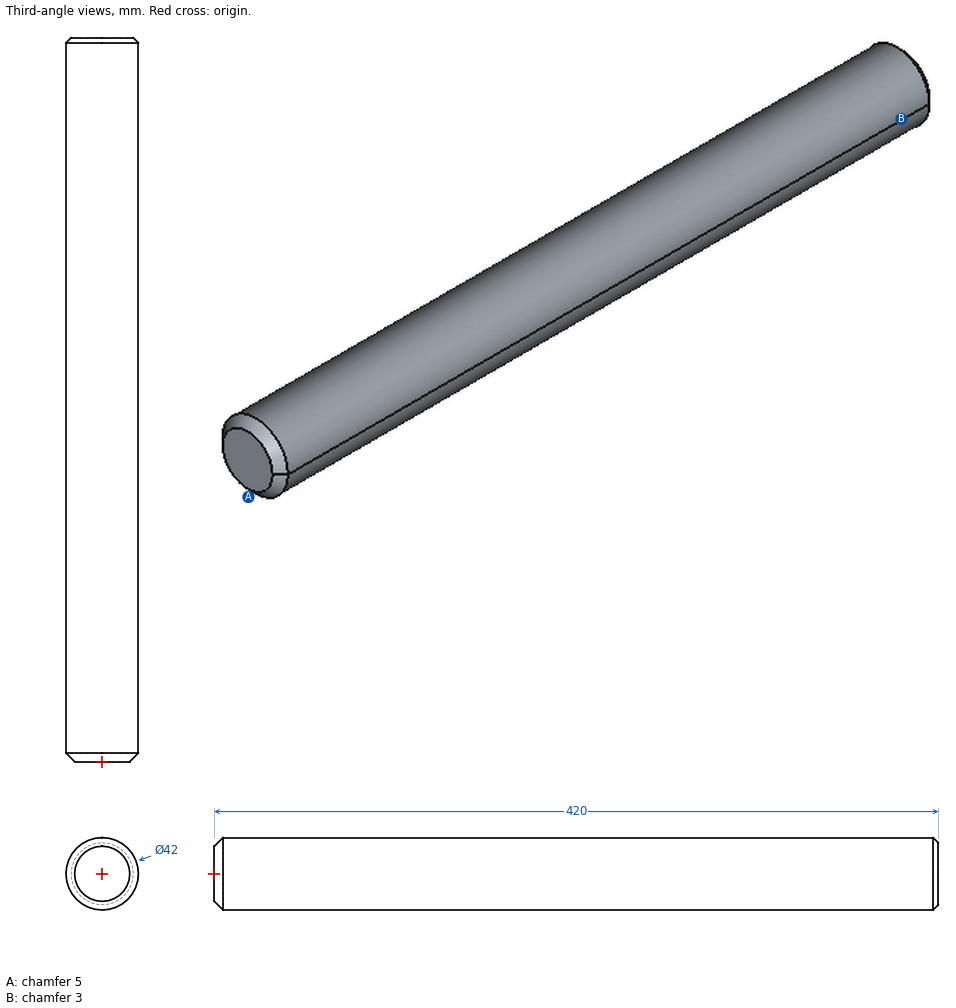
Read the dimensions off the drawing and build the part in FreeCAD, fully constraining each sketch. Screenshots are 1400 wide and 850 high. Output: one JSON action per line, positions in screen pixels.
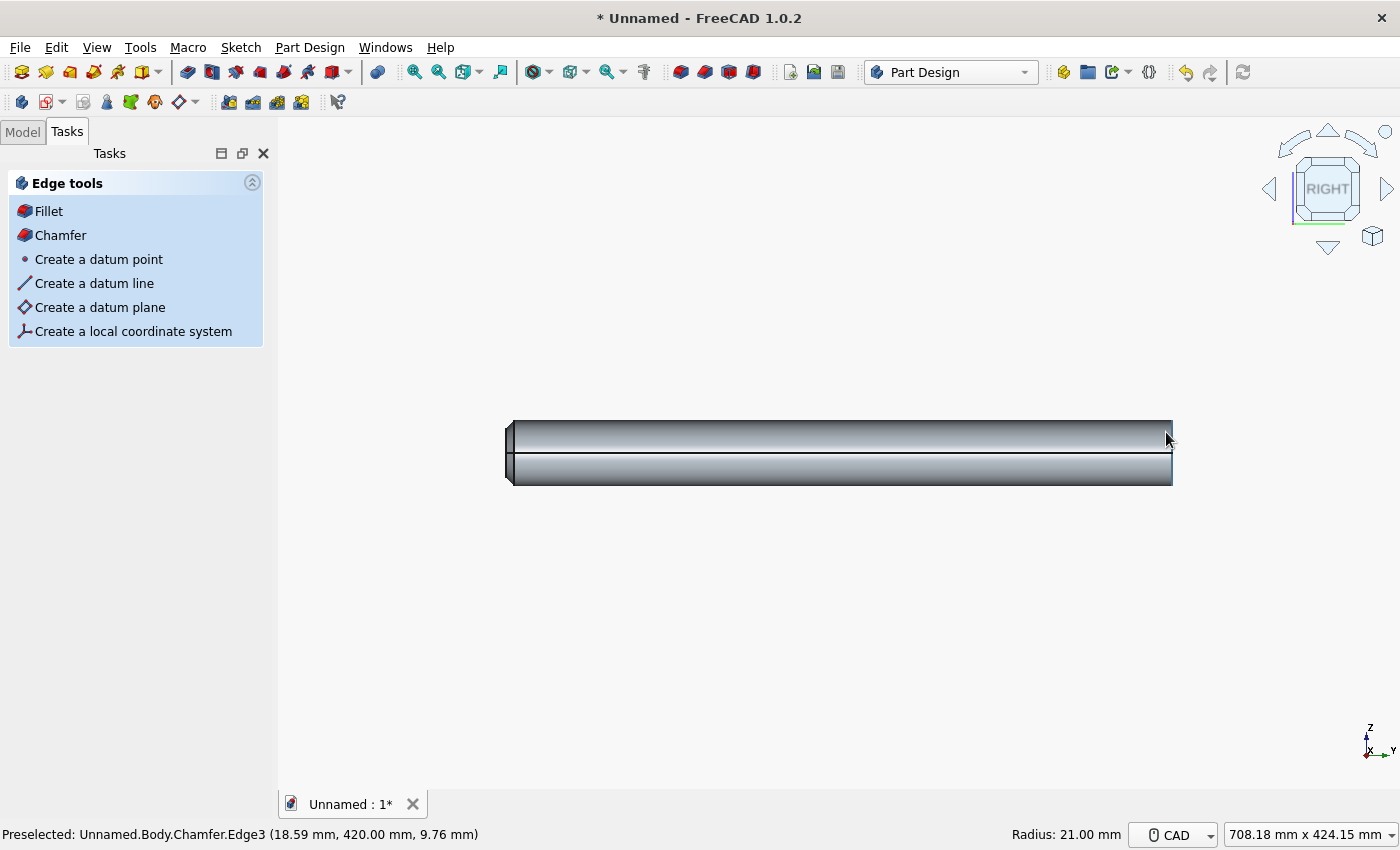
{"action": "left_click", "coordinate": [706, 72]}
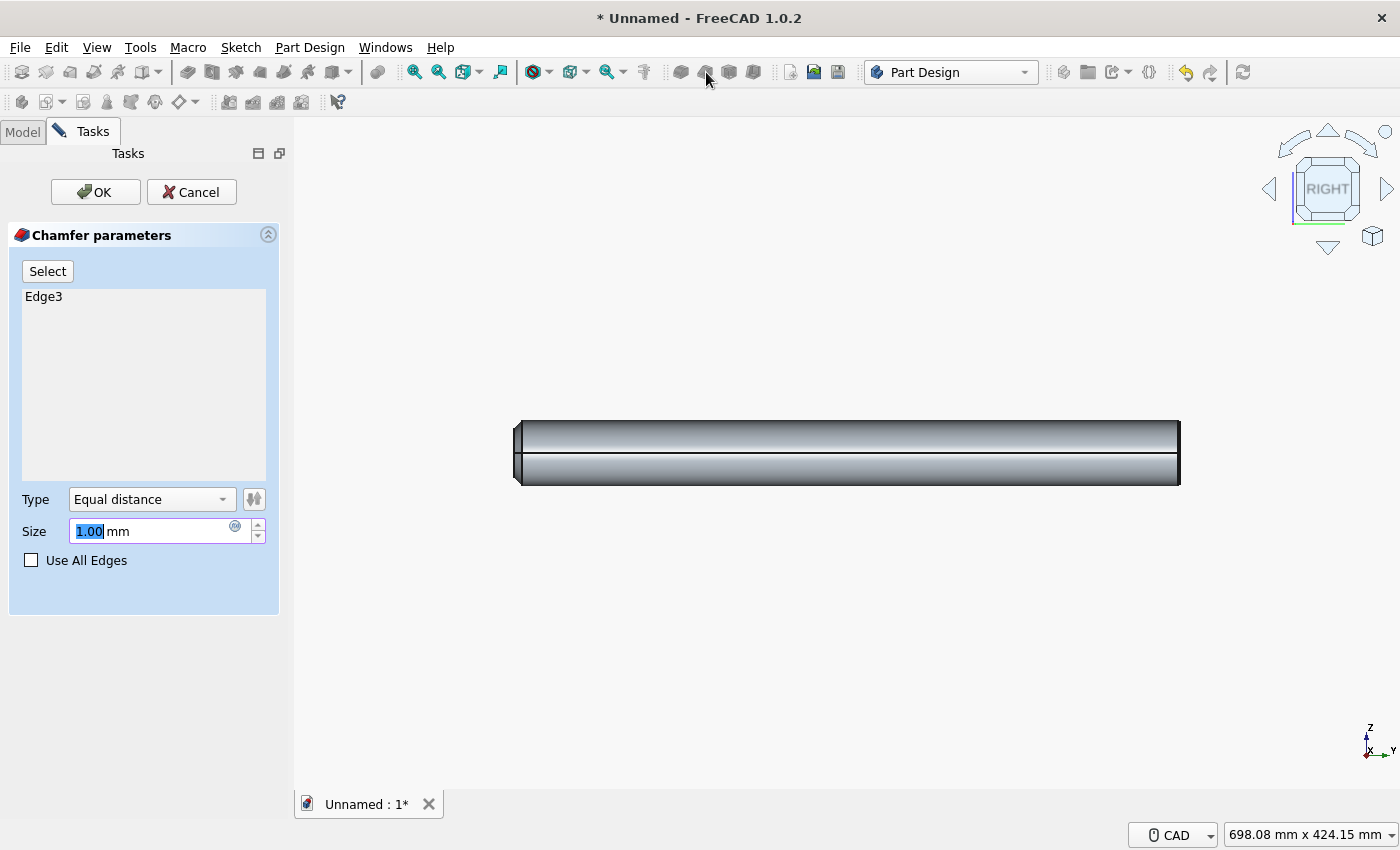
{"action": "type", "text": "3"}
{"action": "key", "text": "Tab"}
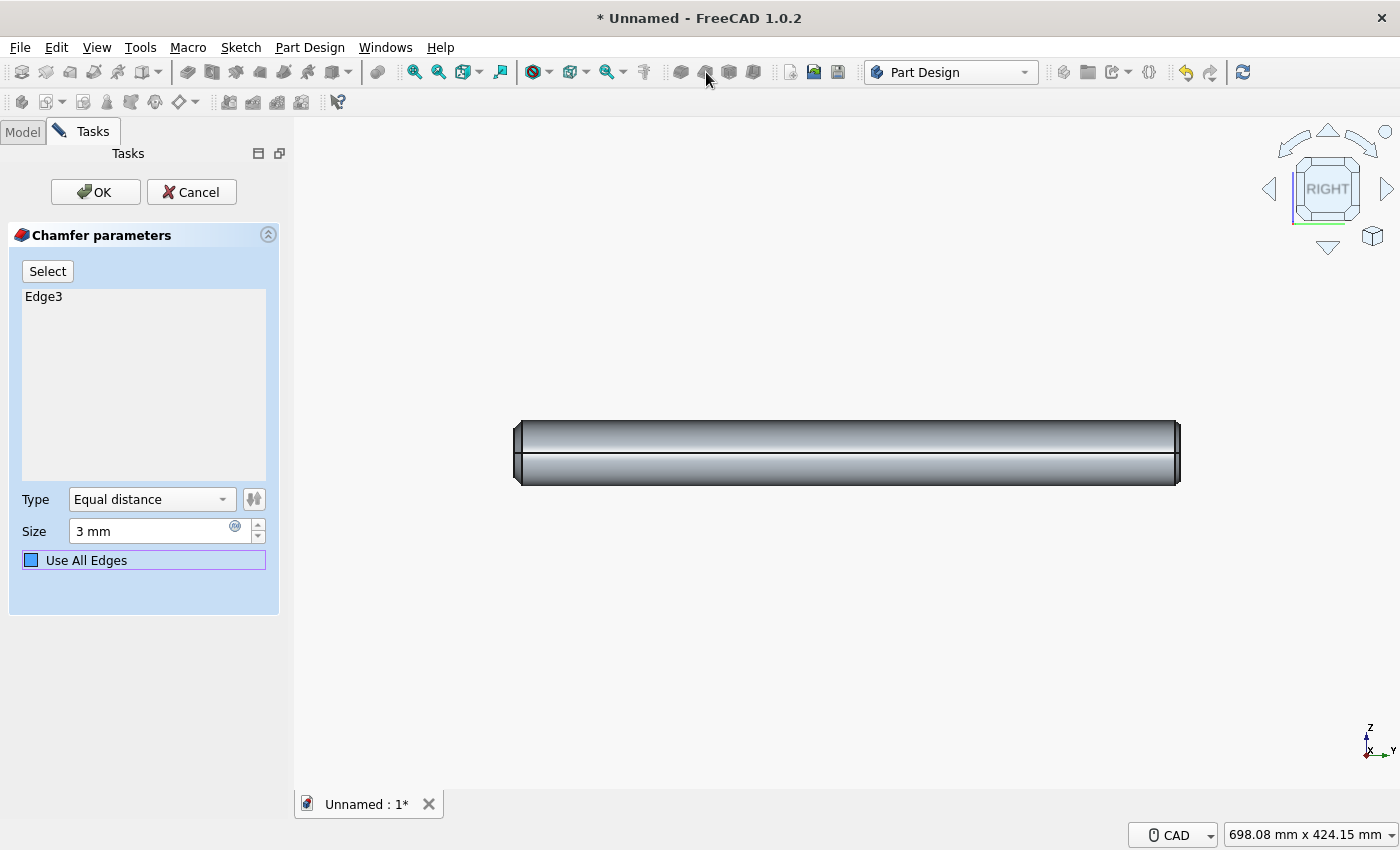
{"action": "left_click", "coordinate": [96, 192]}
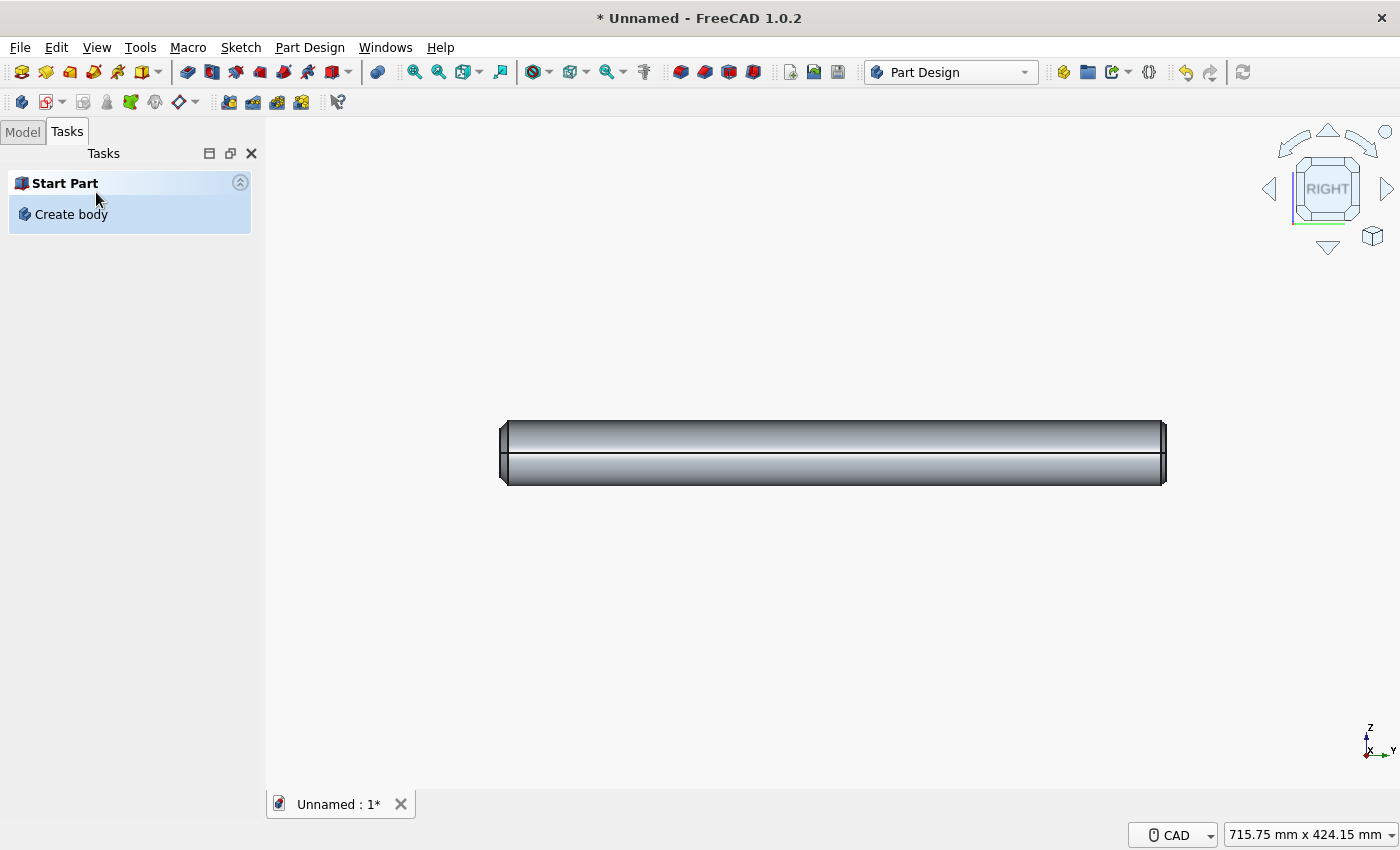
{"action": "key", "text": "0"}